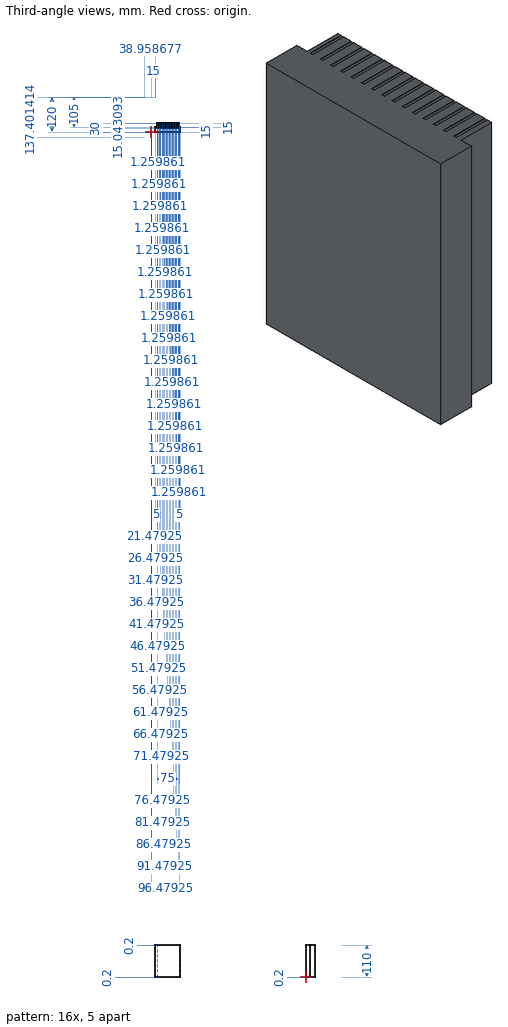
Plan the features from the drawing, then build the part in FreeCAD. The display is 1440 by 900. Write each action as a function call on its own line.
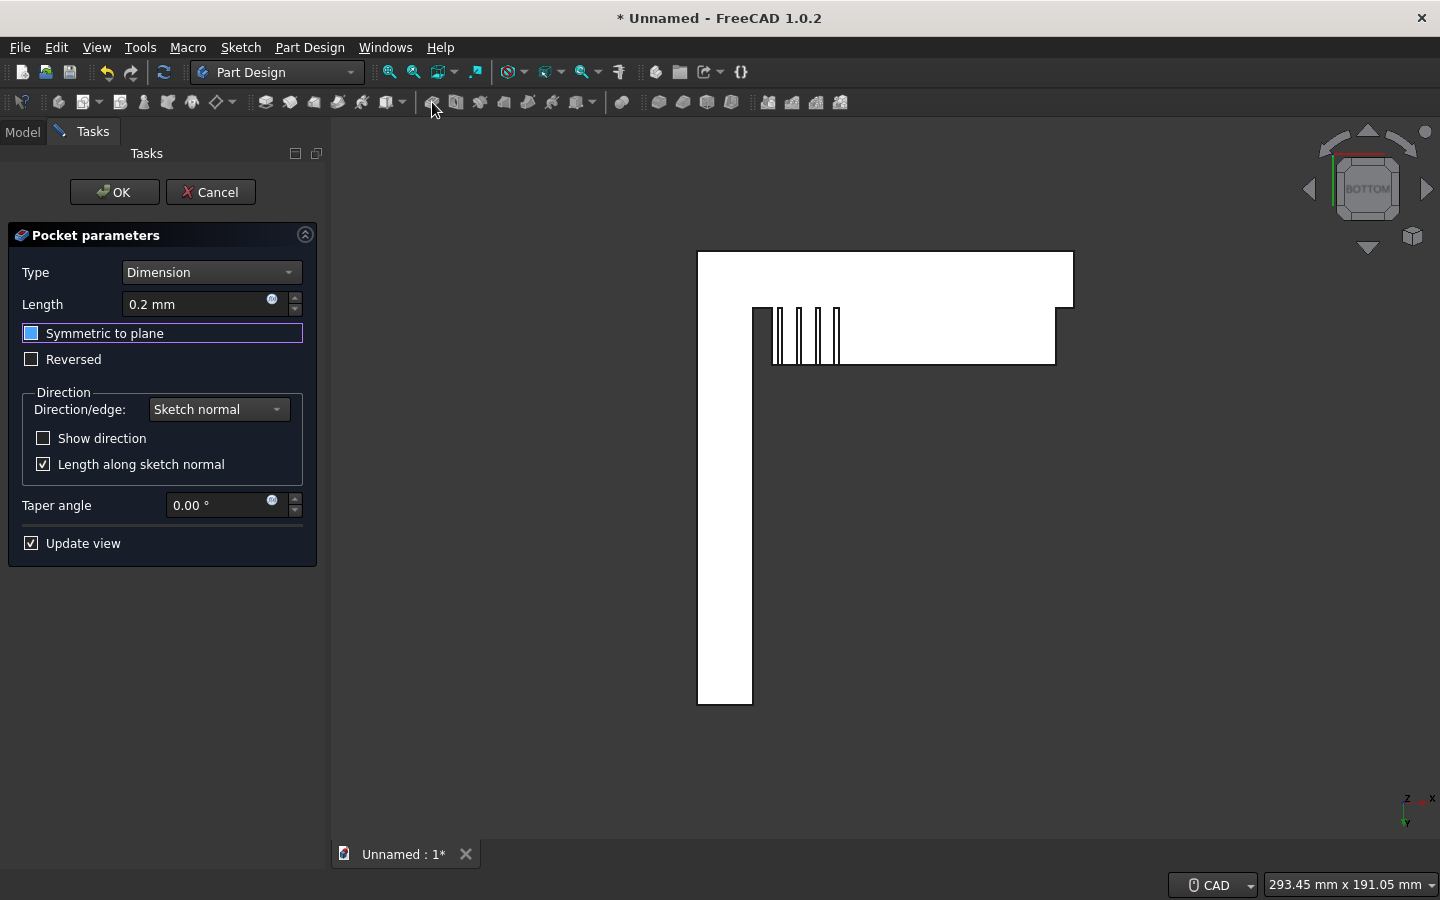
click(115, 192)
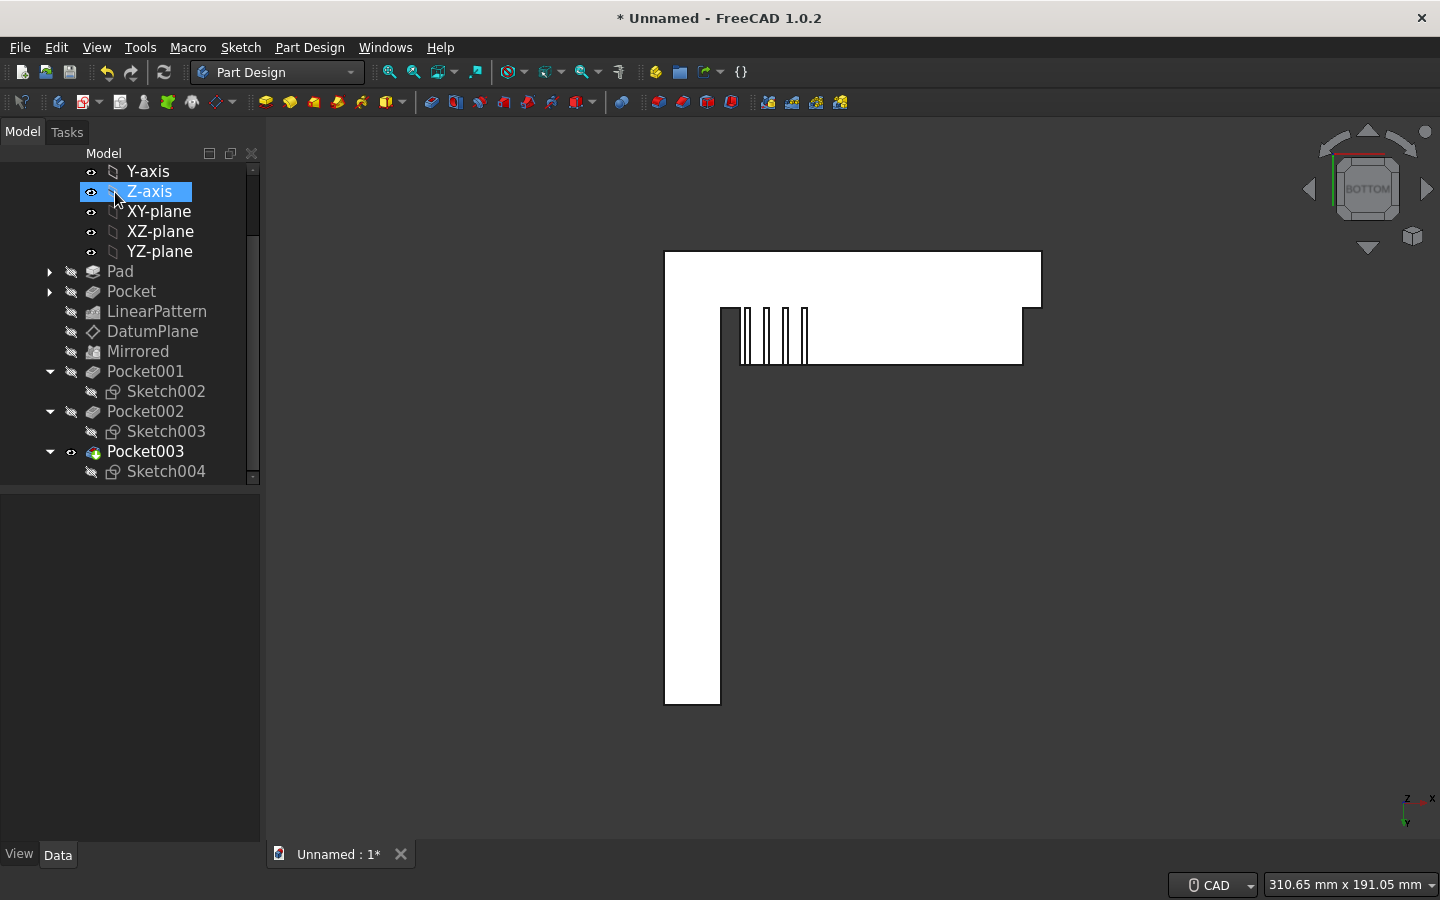
click(84, 102)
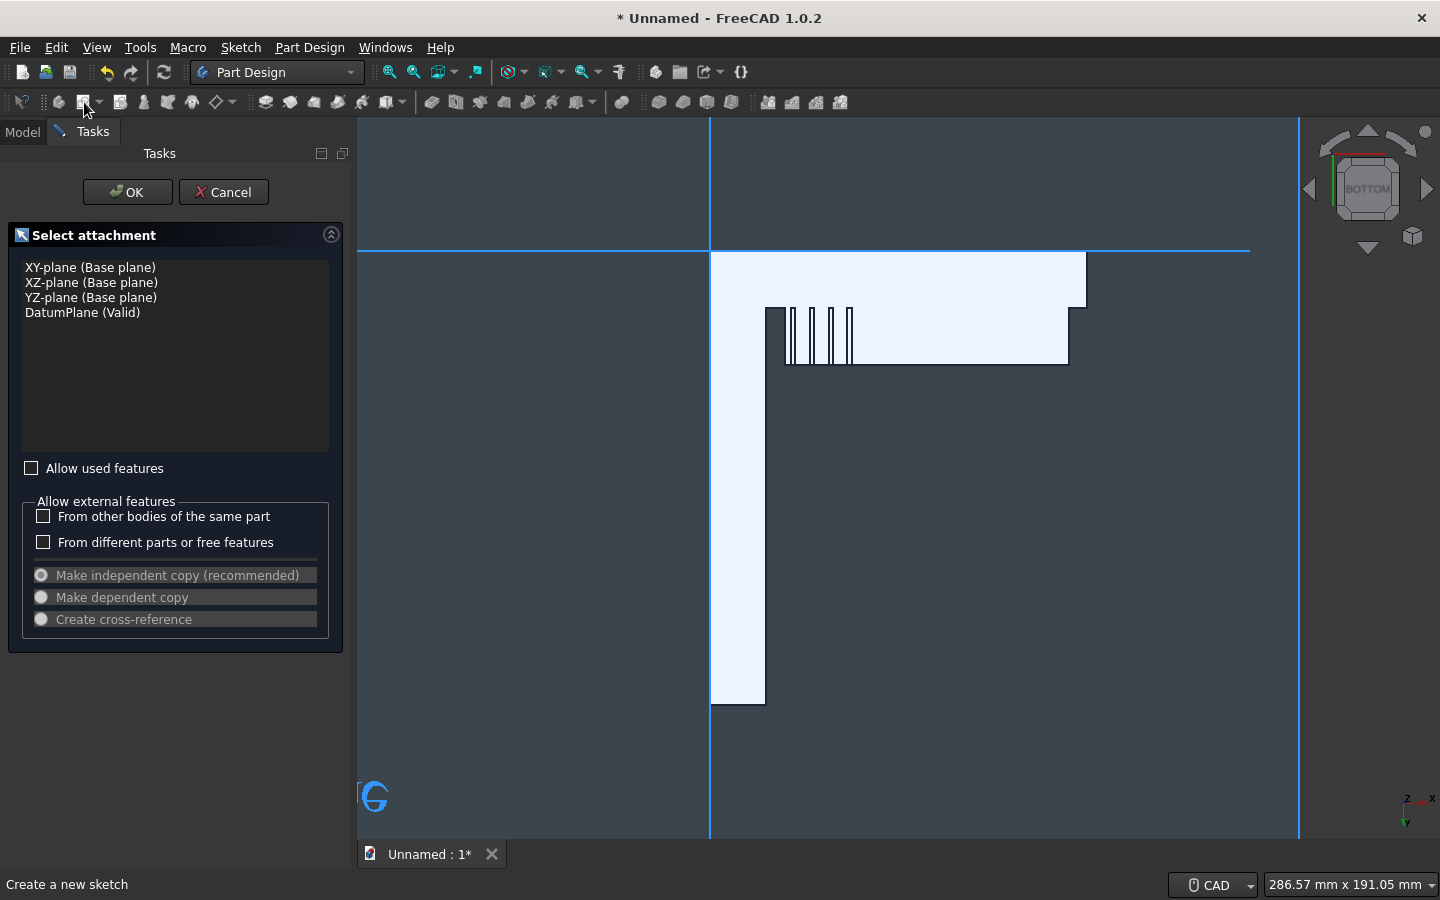
click(82, 268)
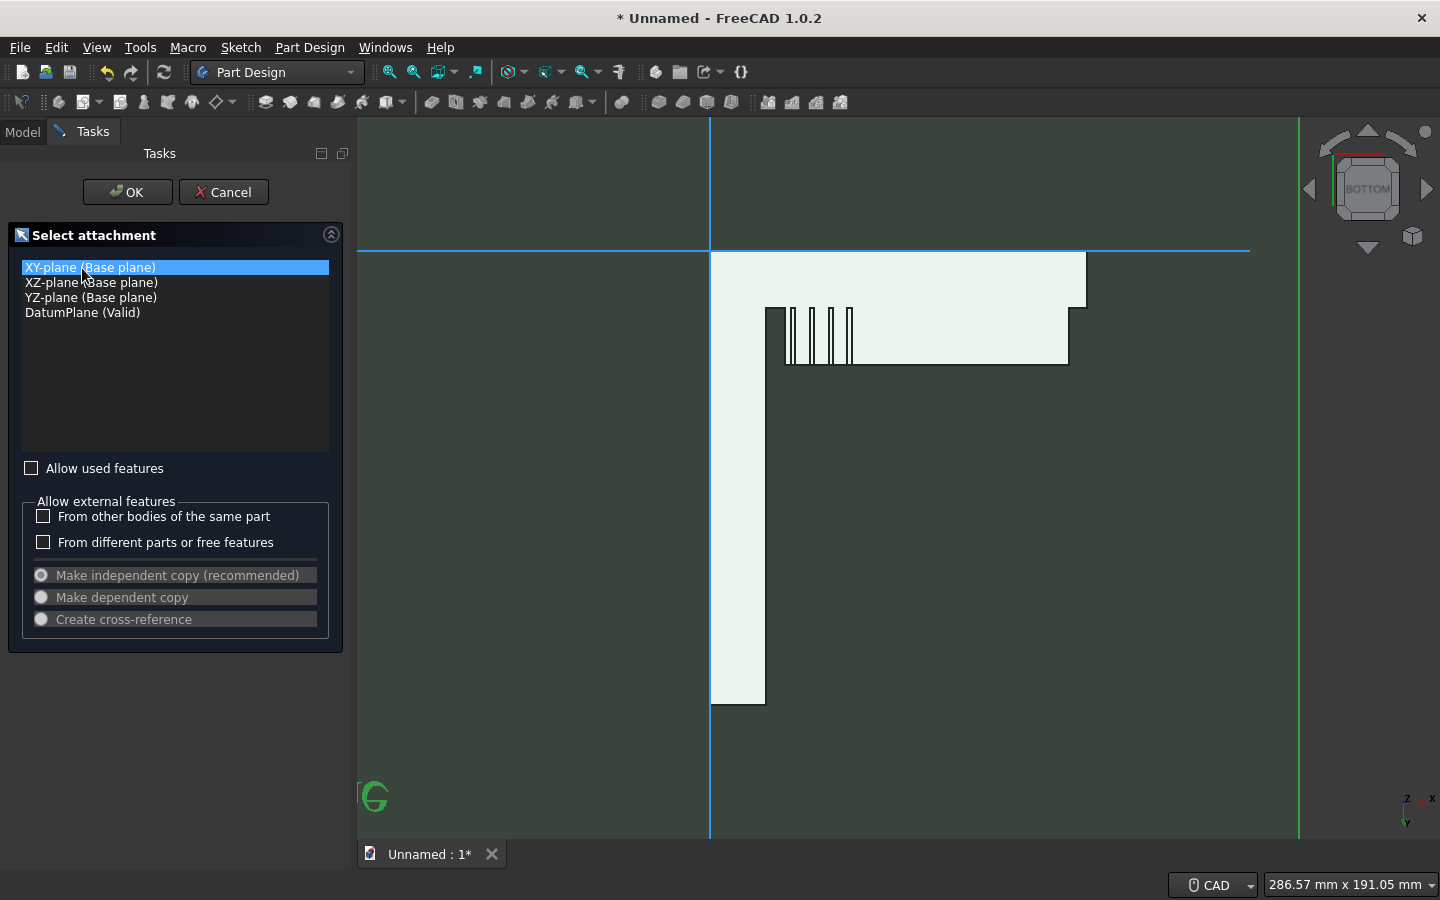
click(128, 192)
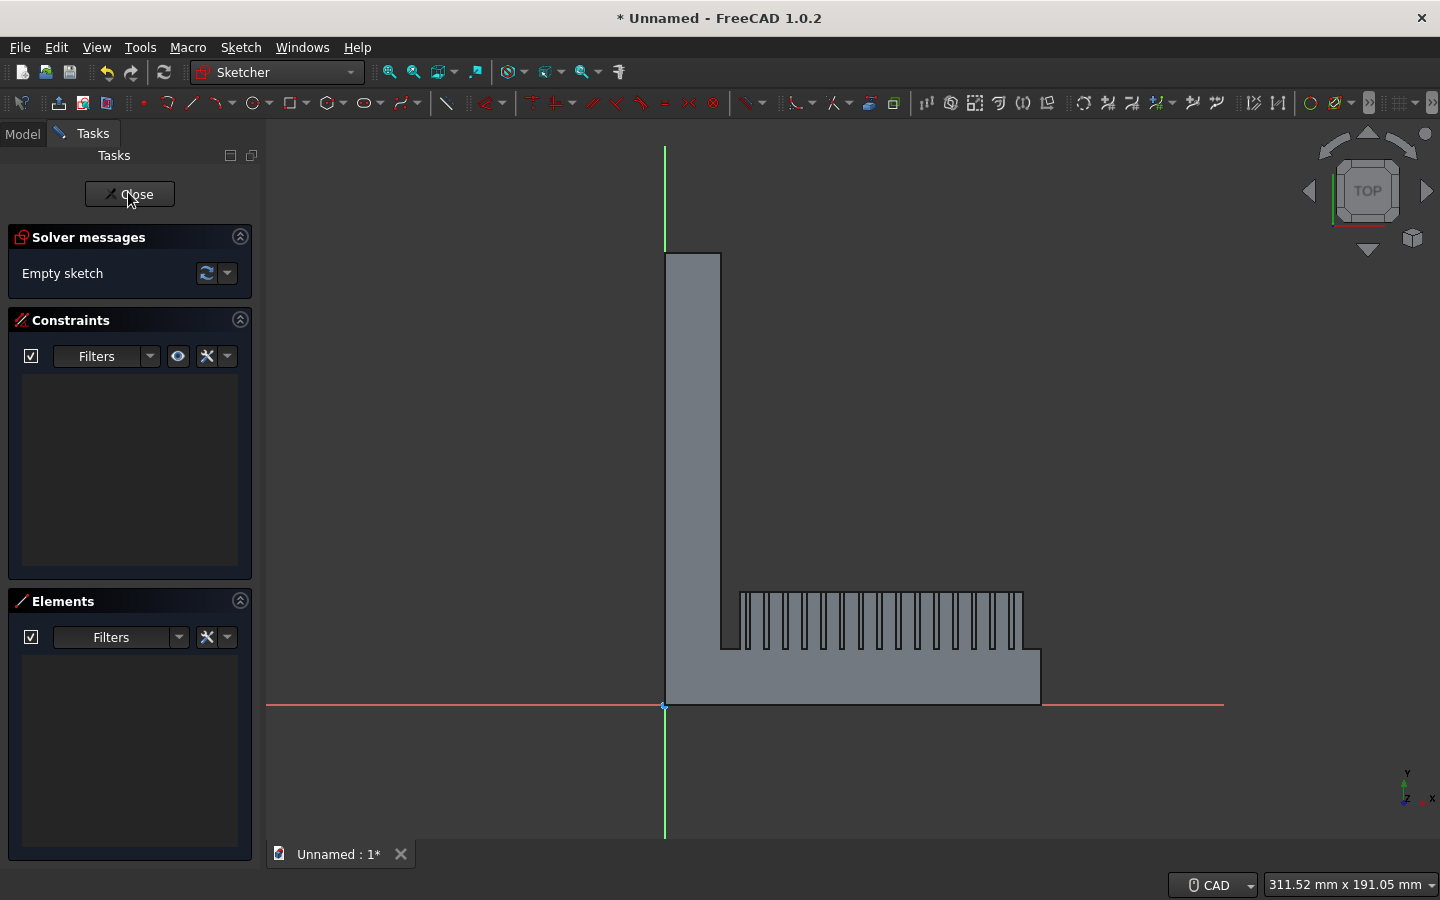
click(108, 104)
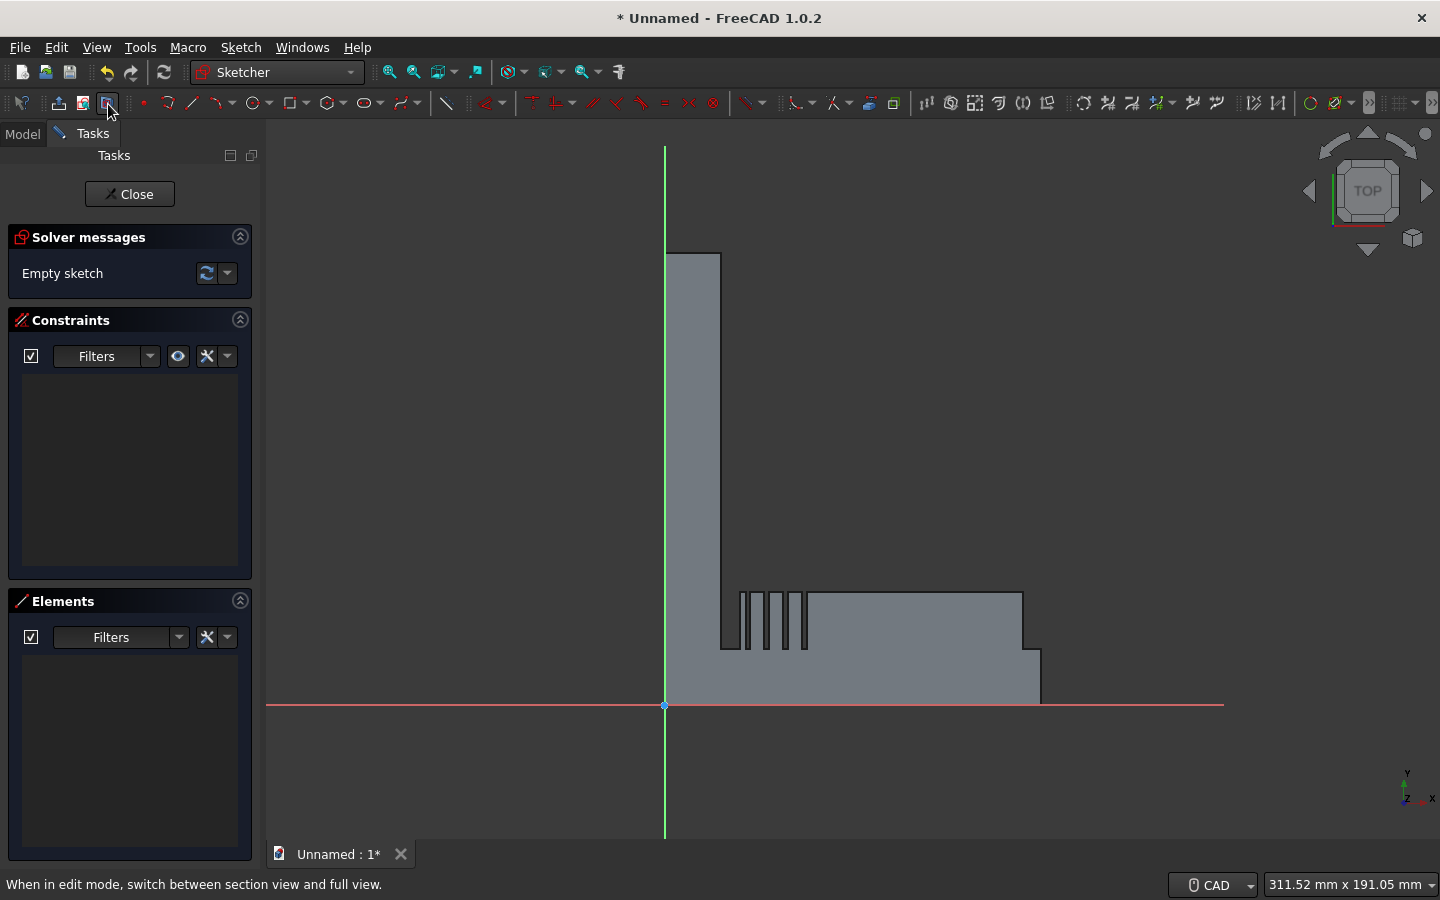
scroll(828, 638, up, 11)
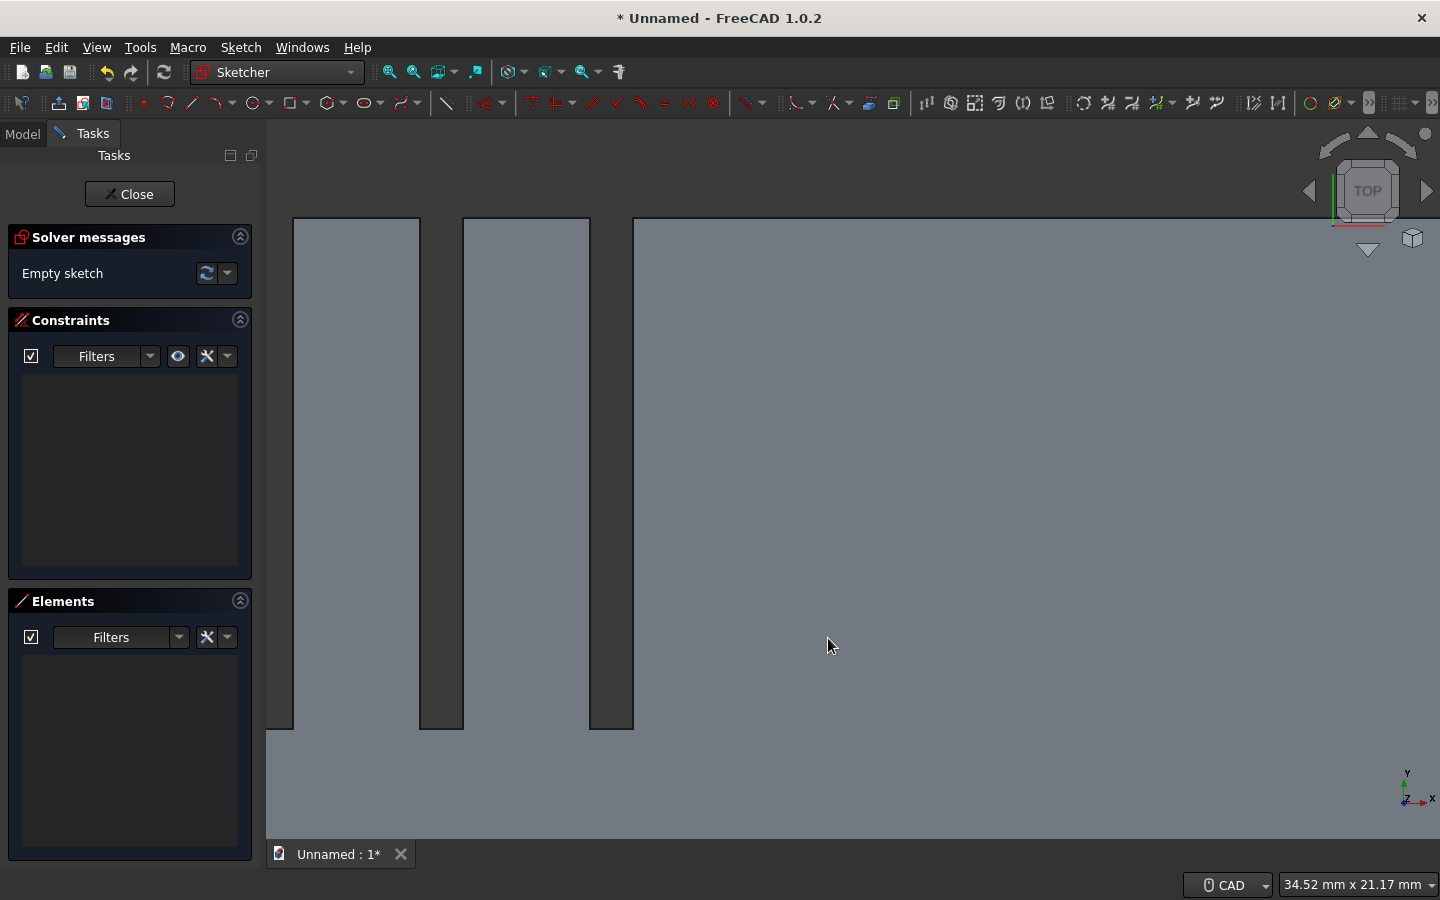
click(290, 104)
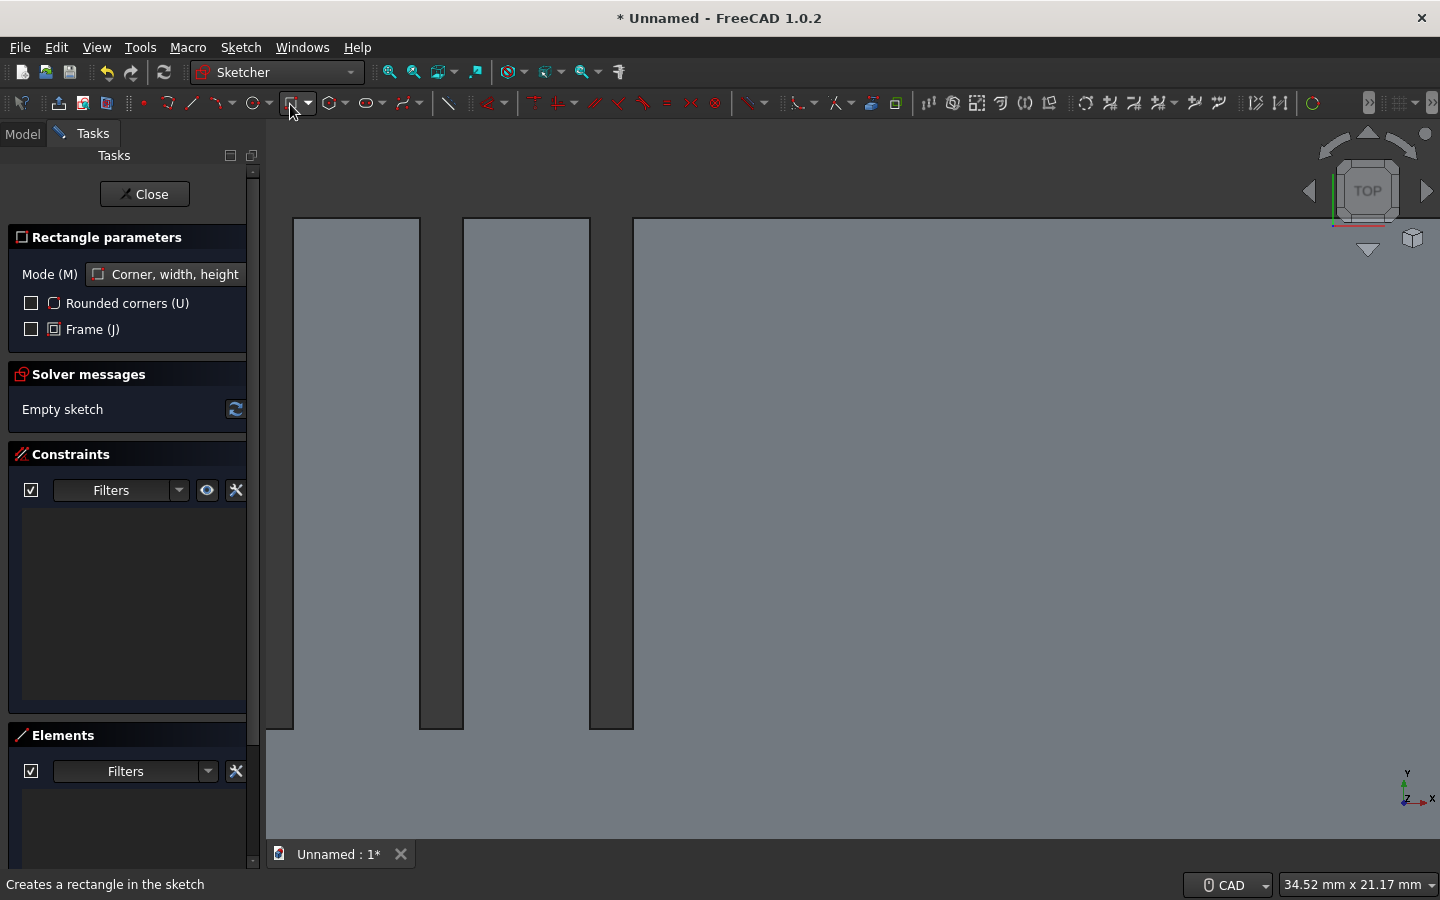
click(760, 218)
click(803, 729)
key(Escape)